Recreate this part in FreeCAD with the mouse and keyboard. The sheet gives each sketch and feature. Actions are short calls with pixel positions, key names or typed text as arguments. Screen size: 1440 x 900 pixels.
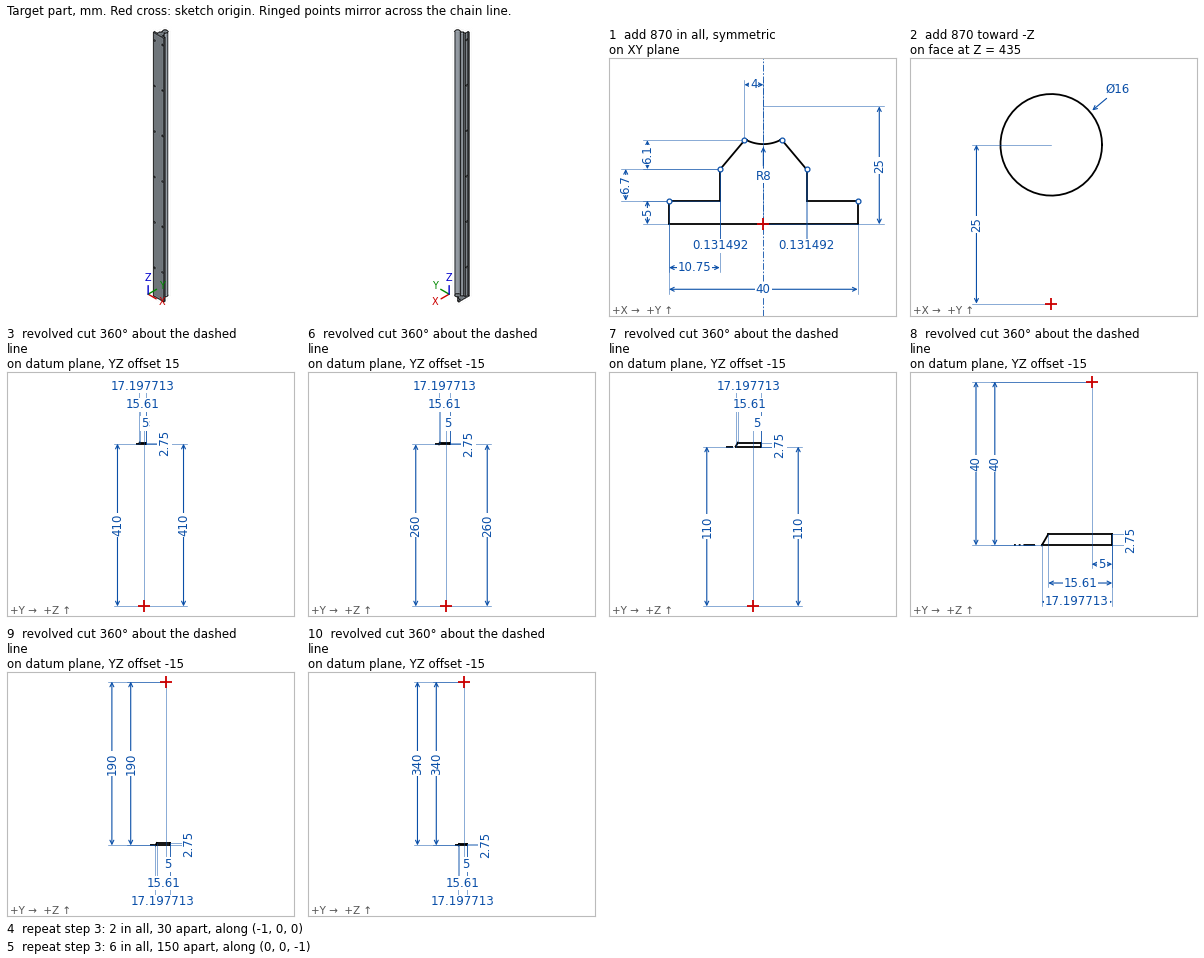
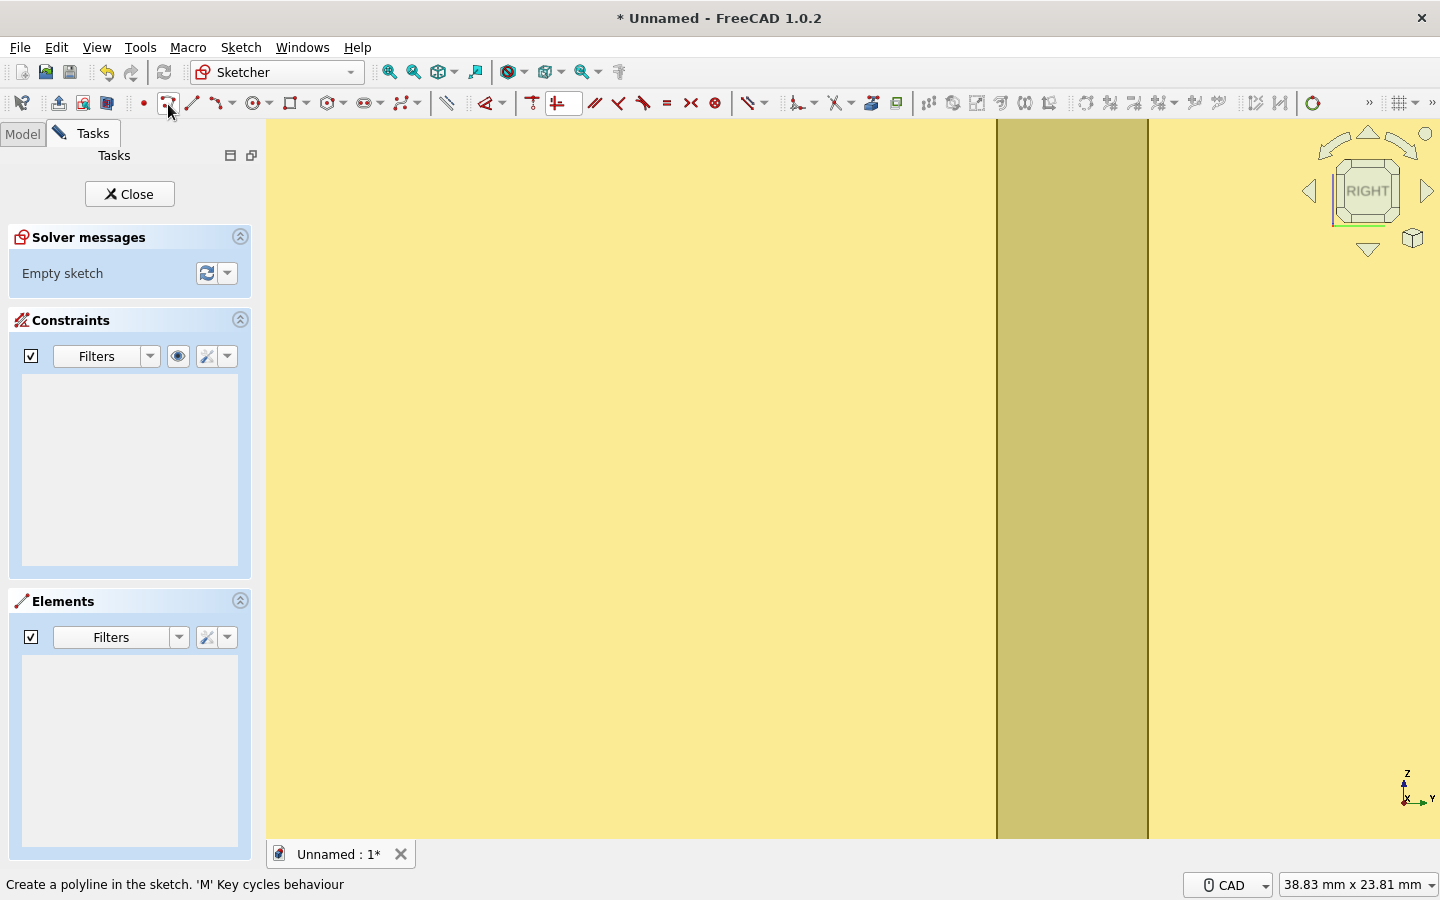
click(1148, 437)
click(676, 437)
click(628, 520)
click(1148, 520)
click(1148, 438)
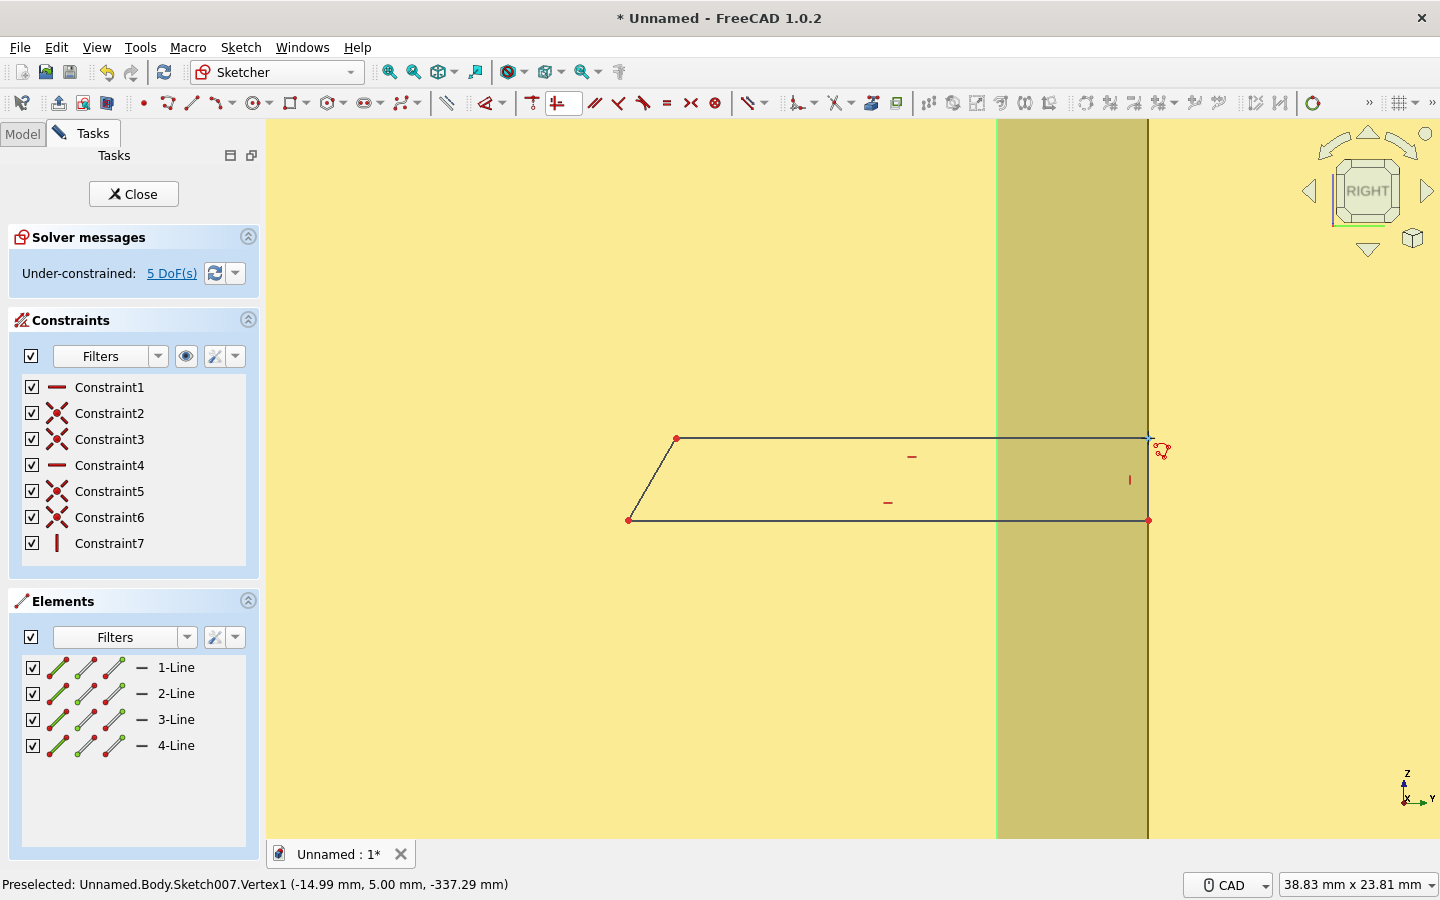
click(192, 104)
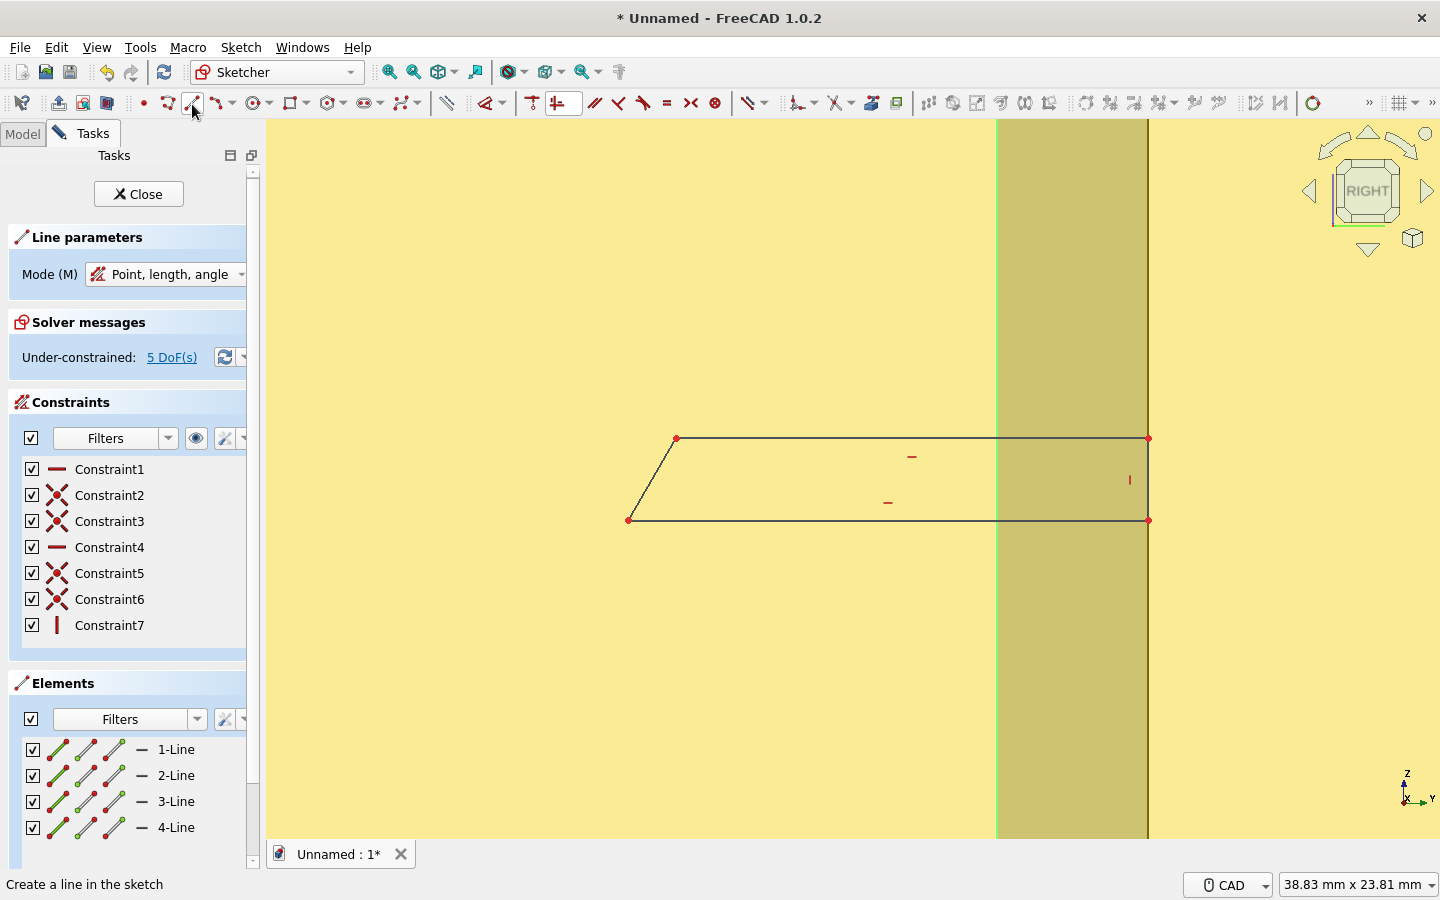
click(576, 520)
click(420, 520)
key(Escape)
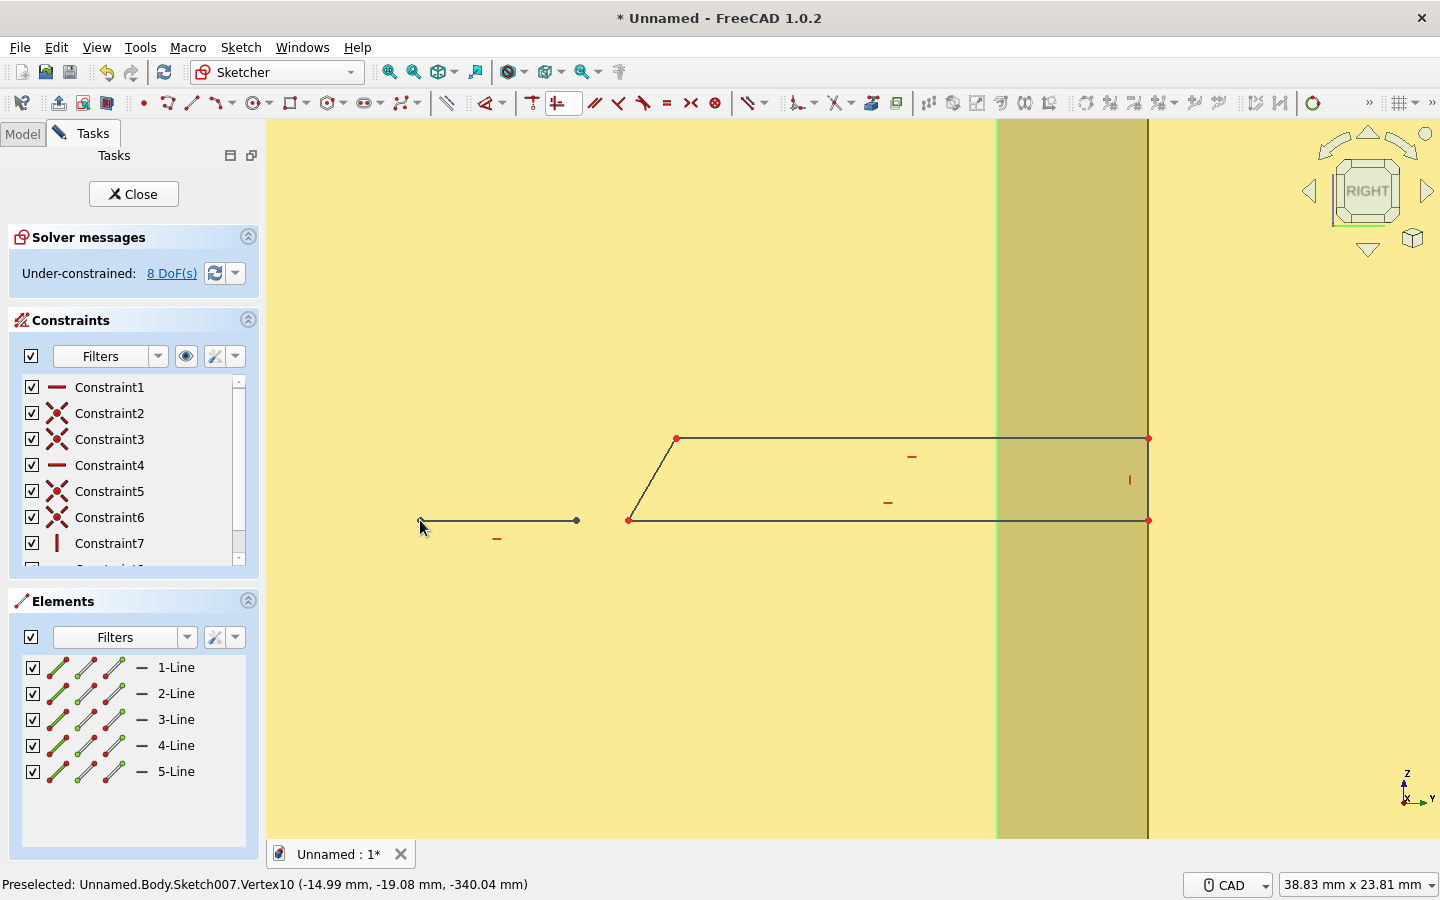
click(529, 521)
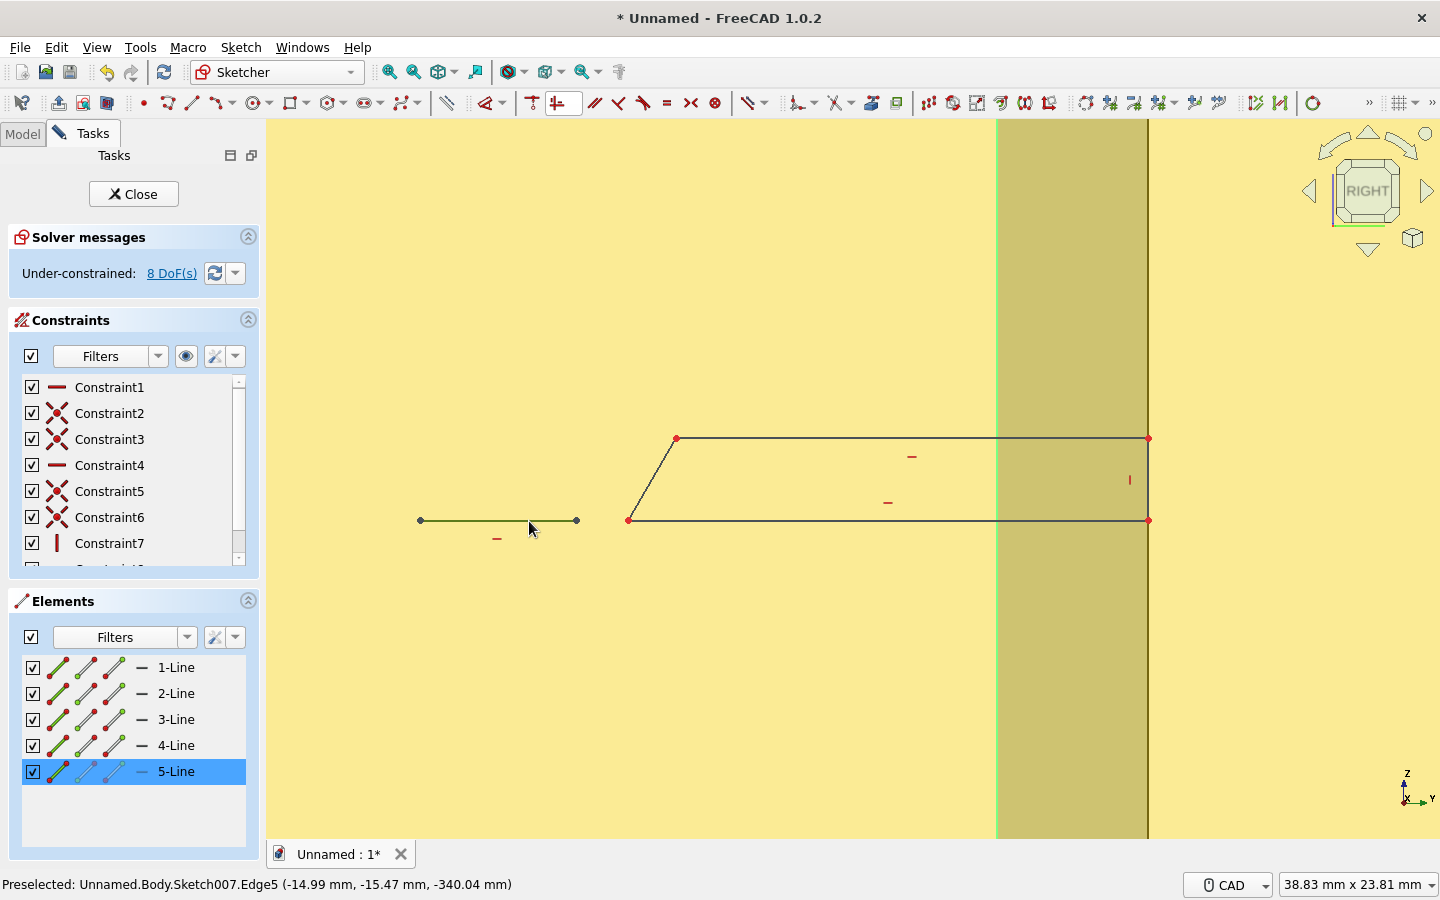
key(g)
key(n)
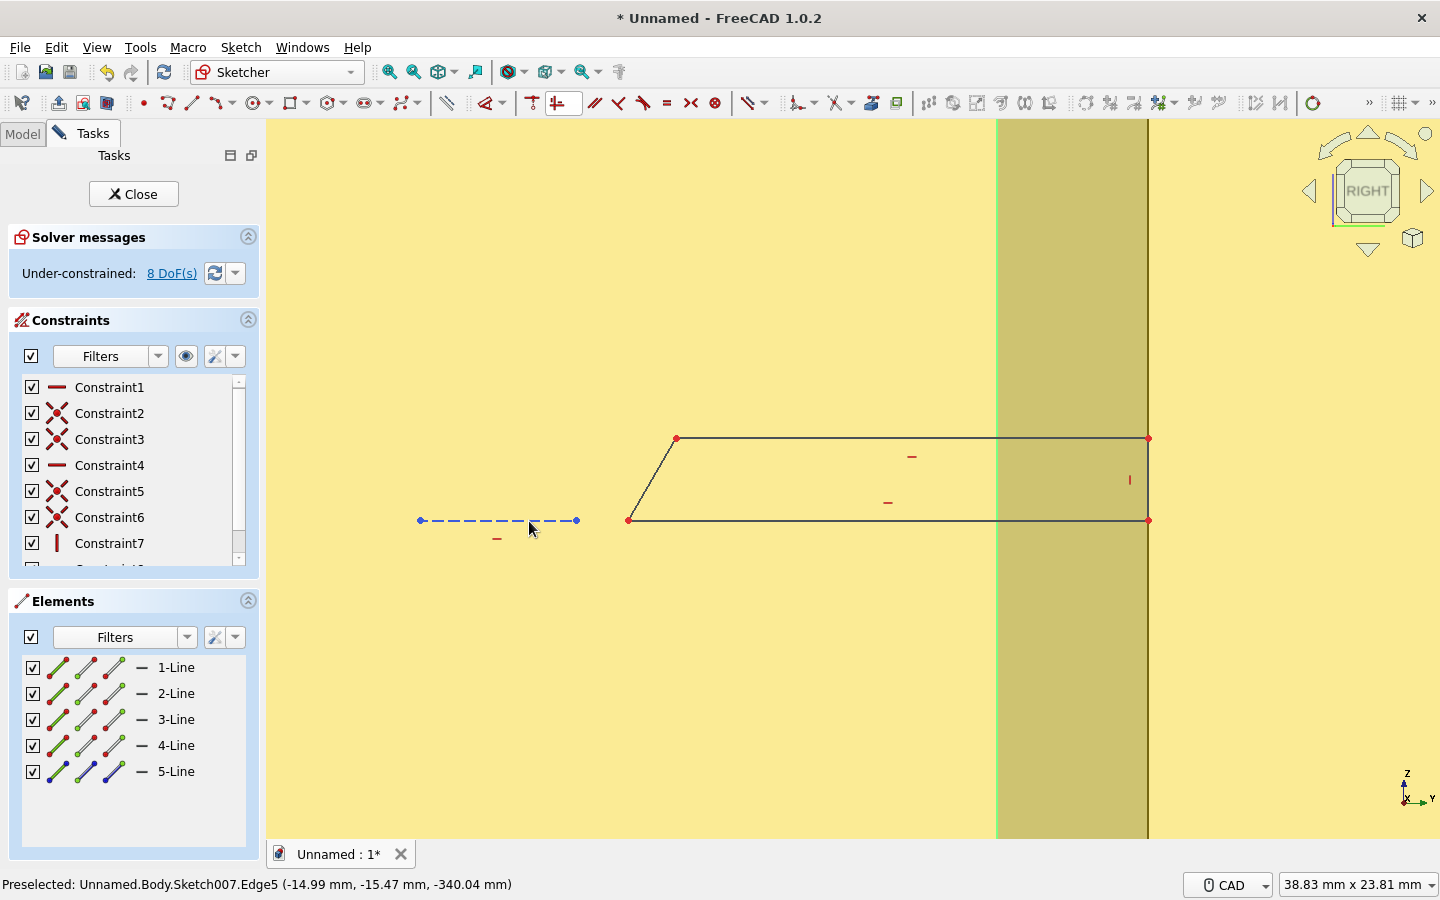
click(486, 104)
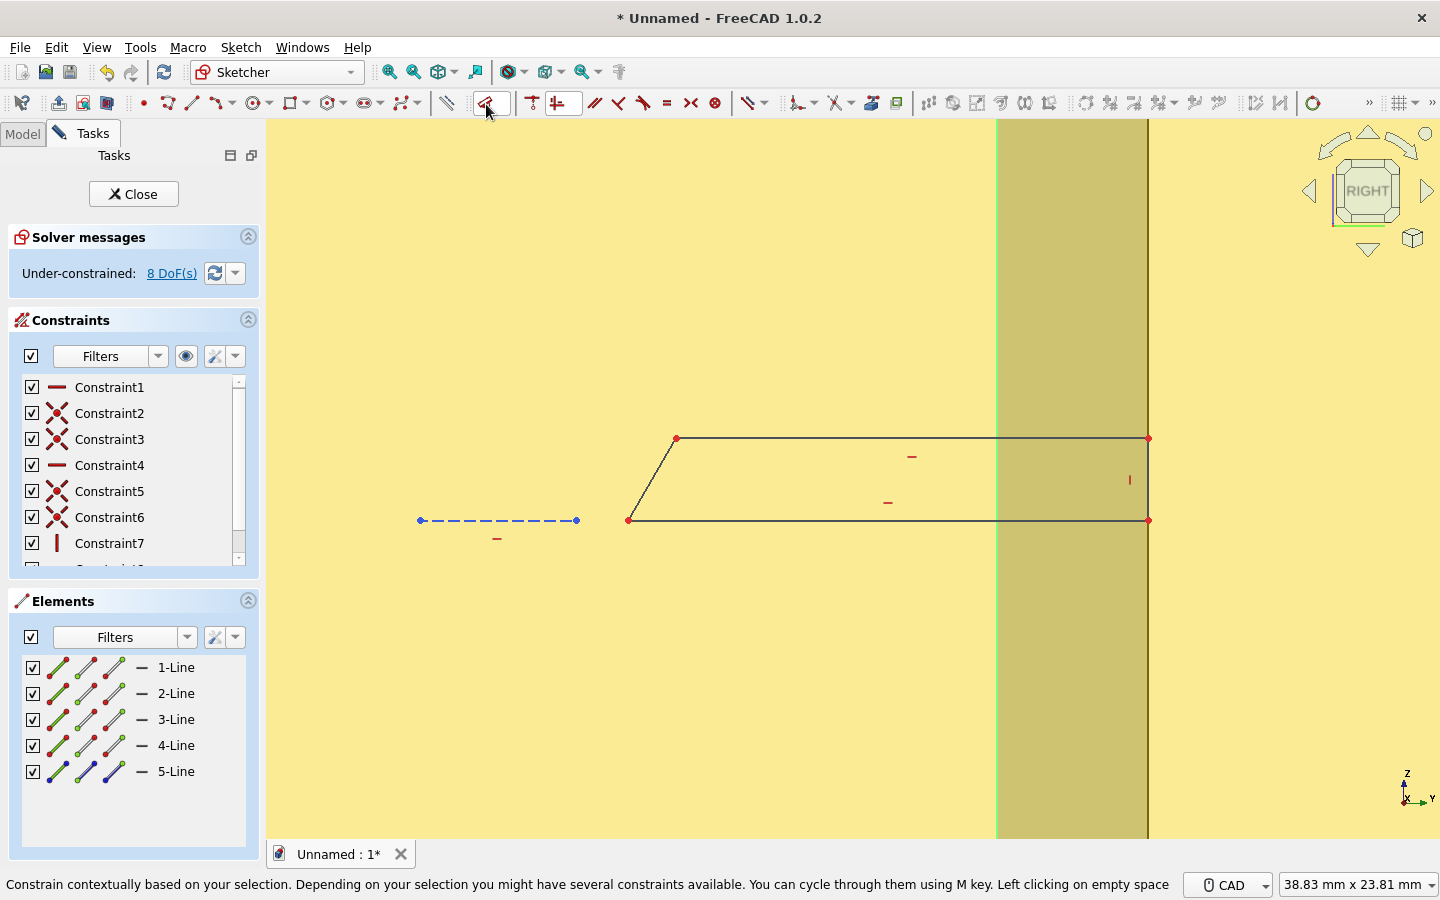
click(1148, 438)
click(1072, 472)